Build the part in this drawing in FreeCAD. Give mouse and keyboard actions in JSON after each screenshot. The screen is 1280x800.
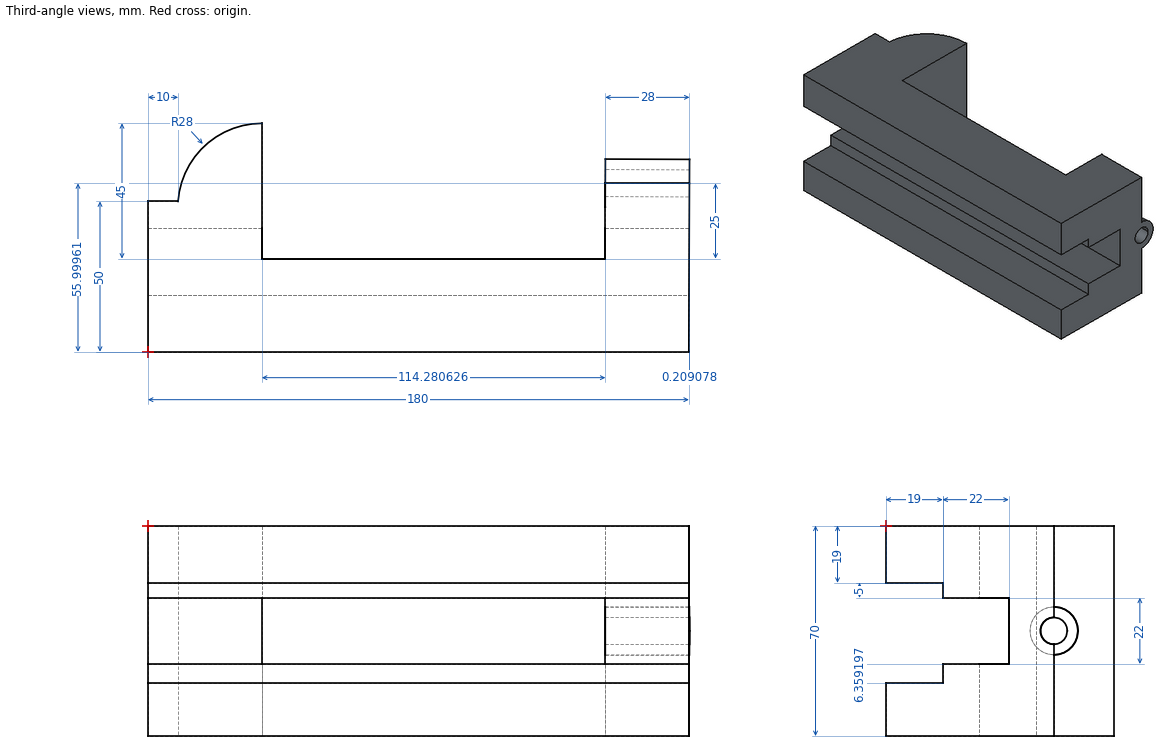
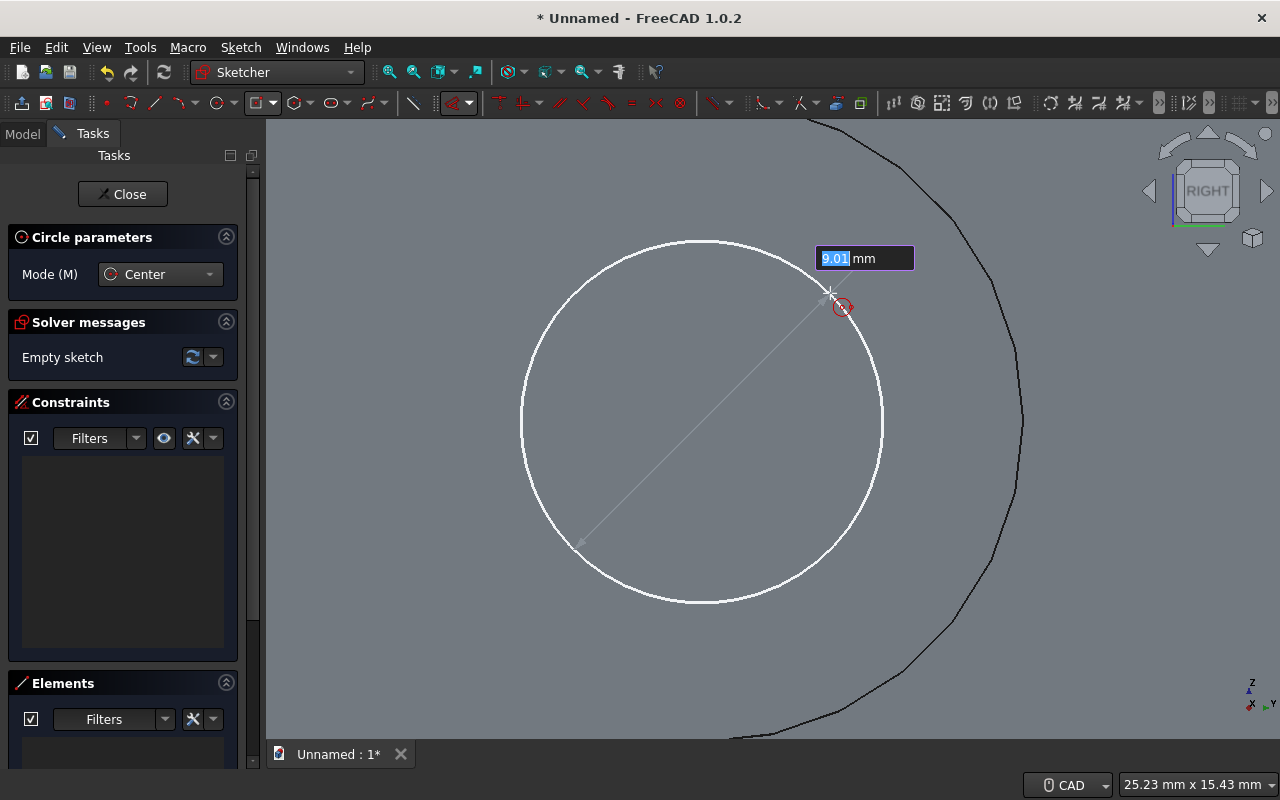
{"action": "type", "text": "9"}
{"action": "key", "text": "Return"}
{"action": "key", "text": "Escape"}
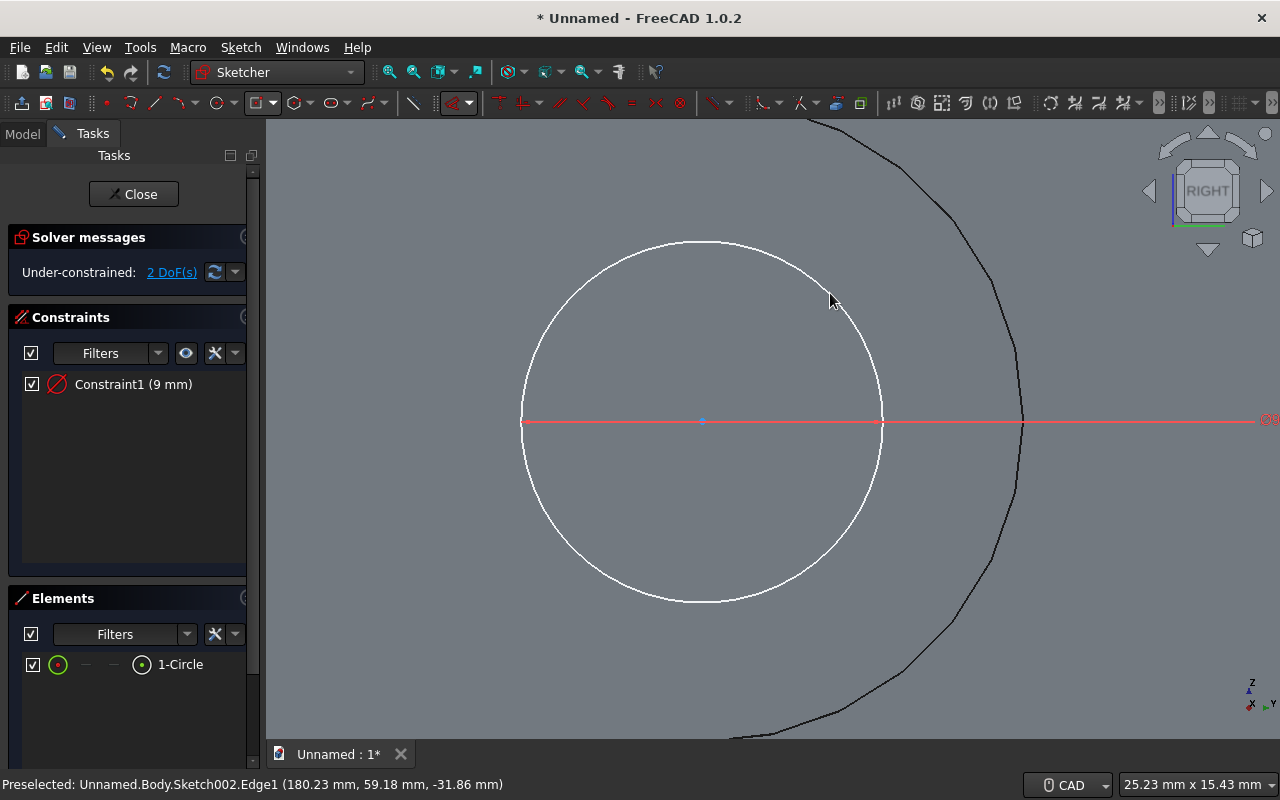
{"action": "left_click", "coordinate": [702, 422]}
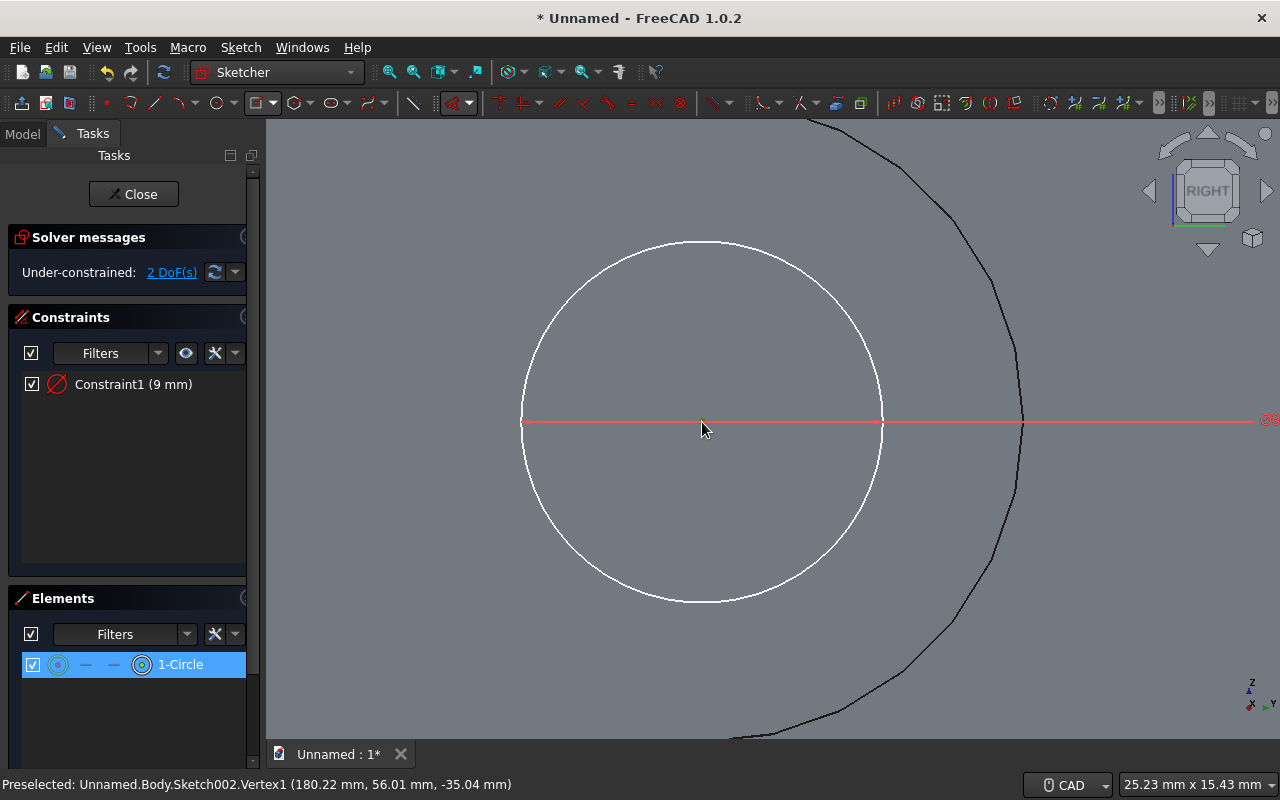
{"action": "key", "text": "i"}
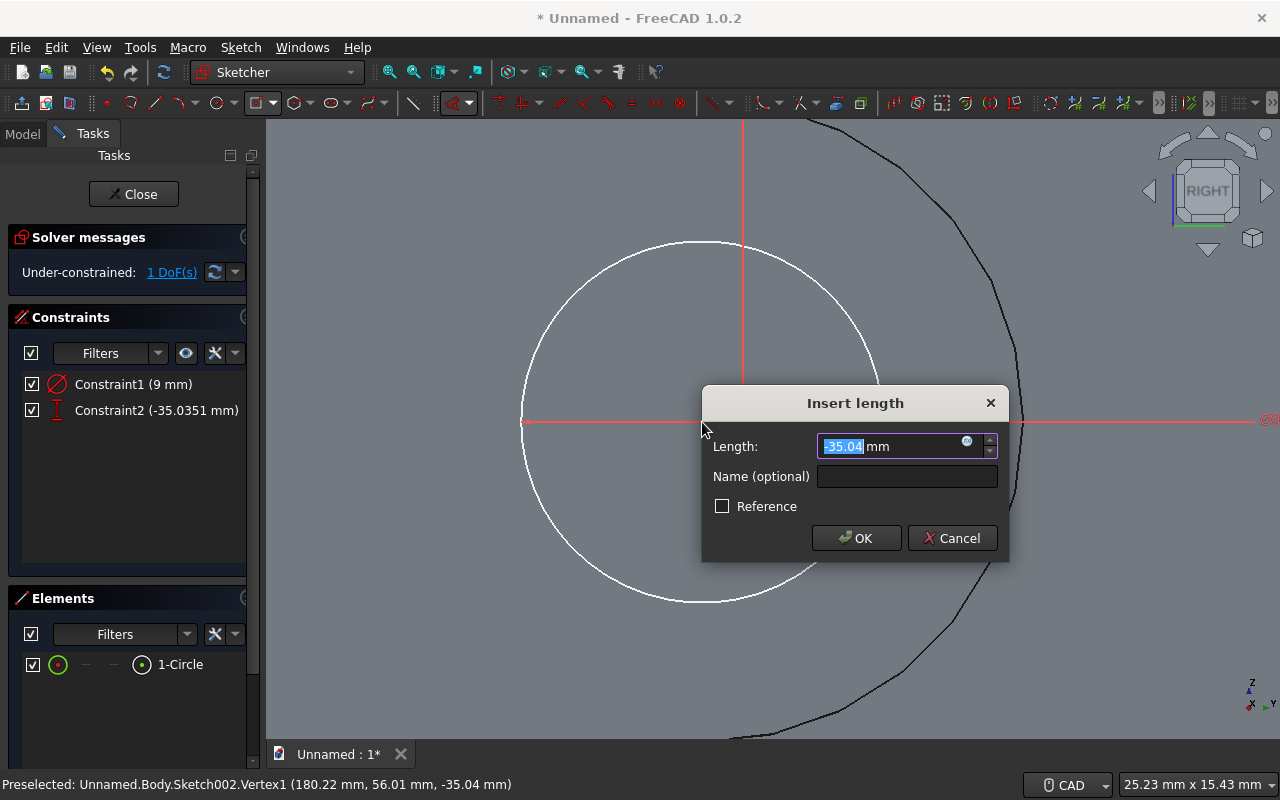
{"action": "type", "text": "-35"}
{"action": "key", "text": "Return"}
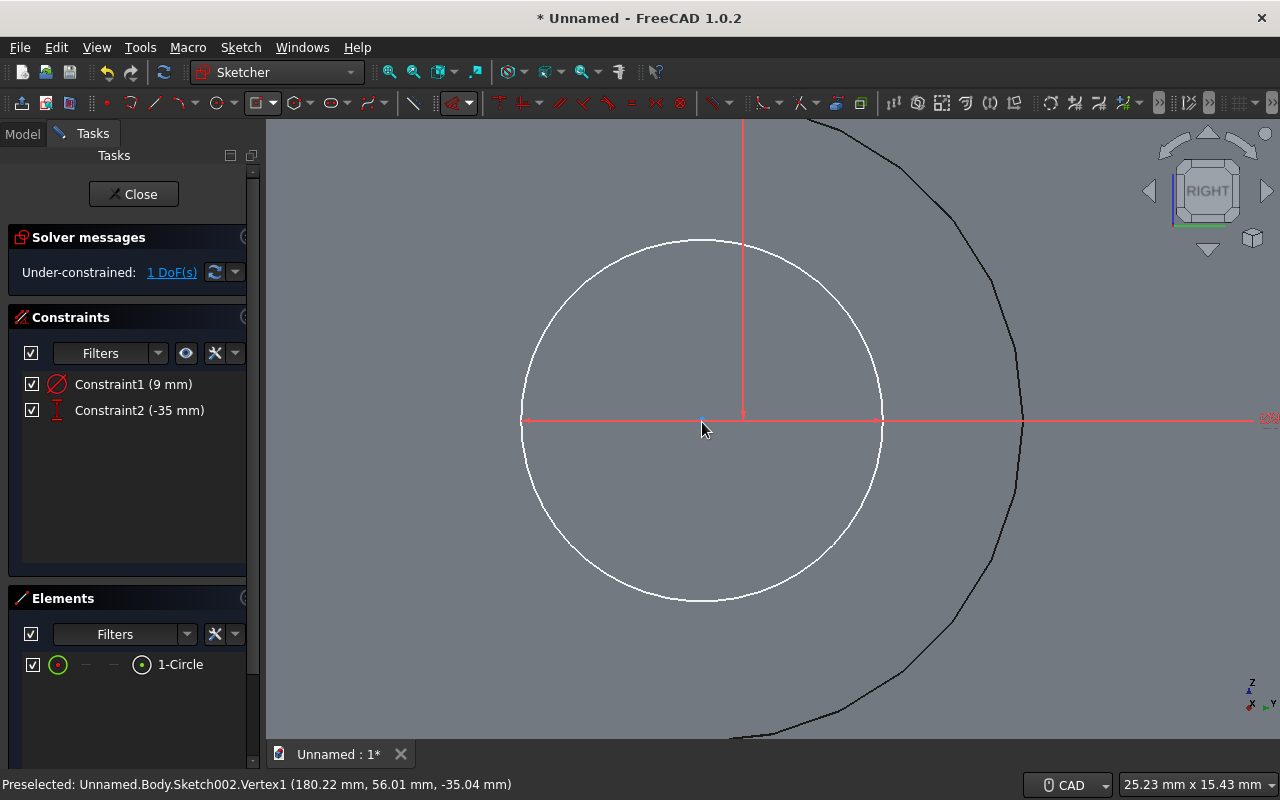
{"action": "left_click", "coordinate": [702, 421]}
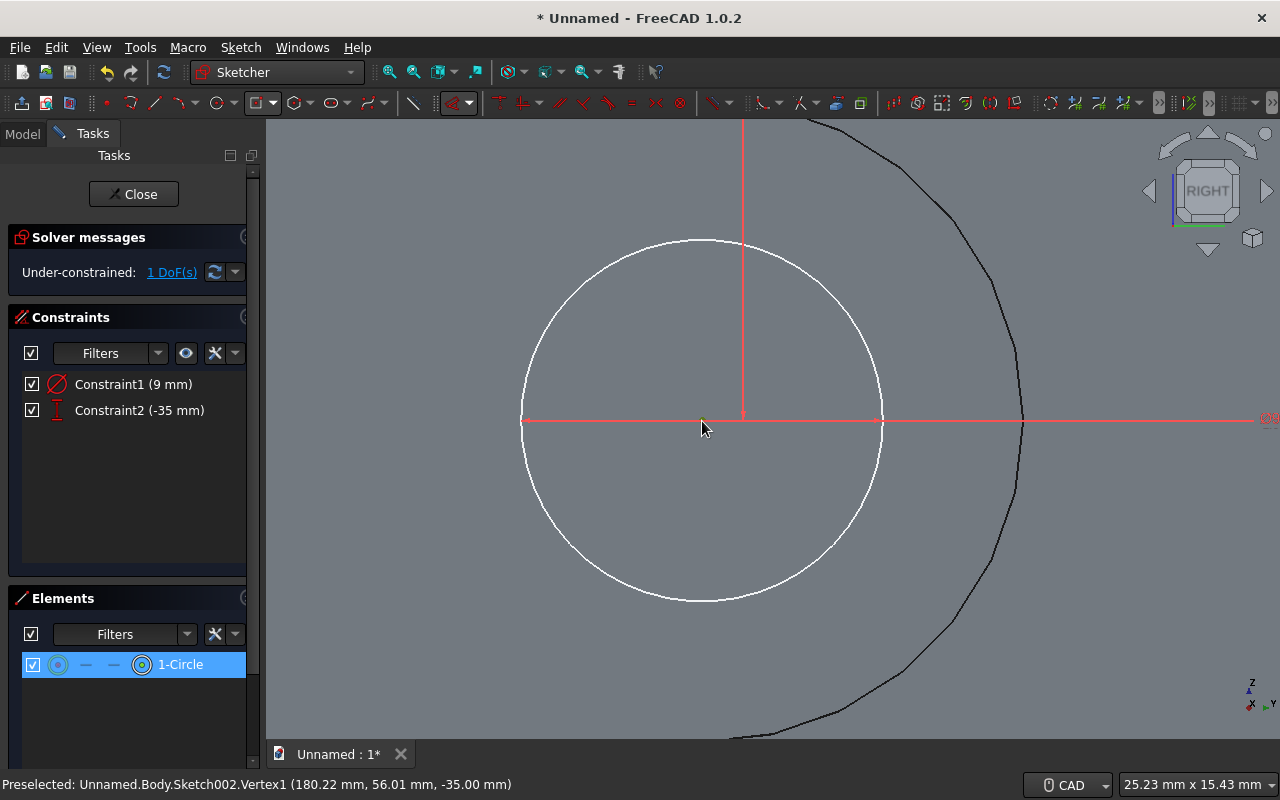
{"action": "left_click", "coordinate": [472, 104]}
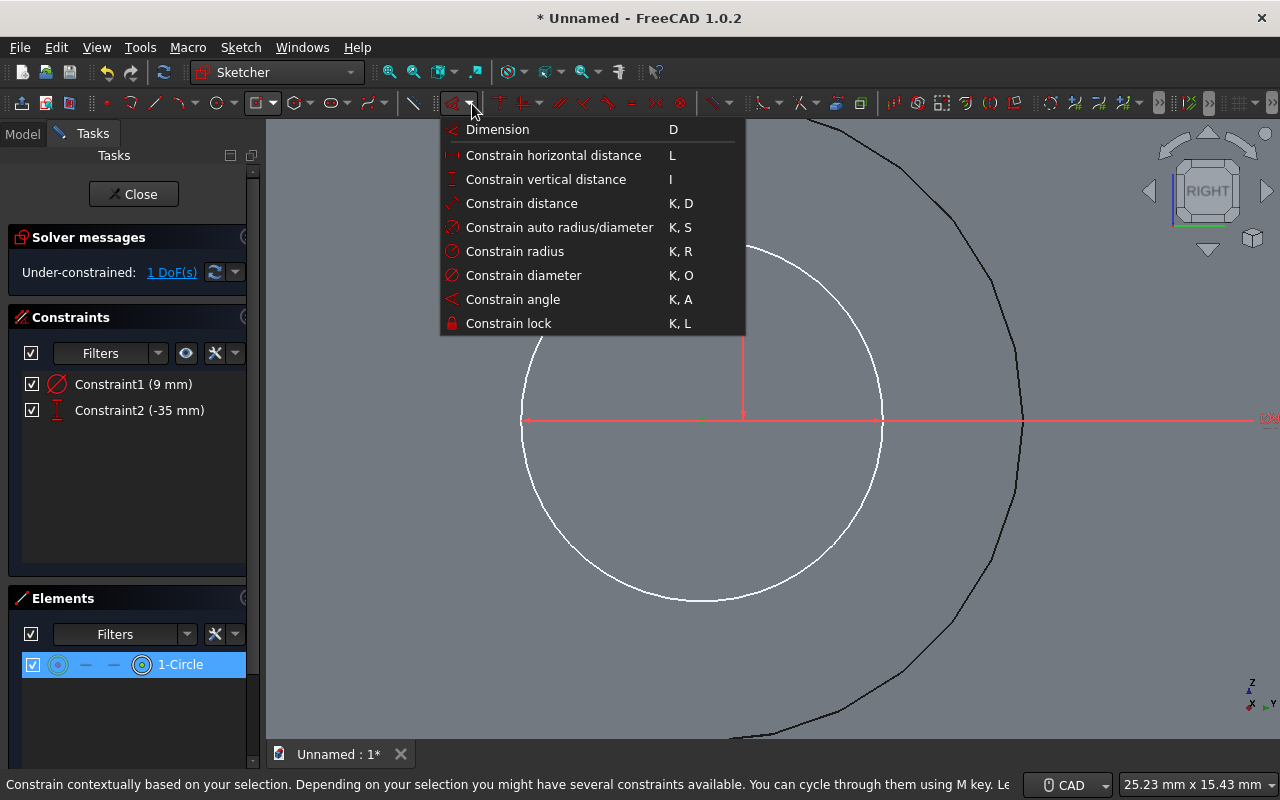
{"action": "left_click", "coordinate": [593, 155]}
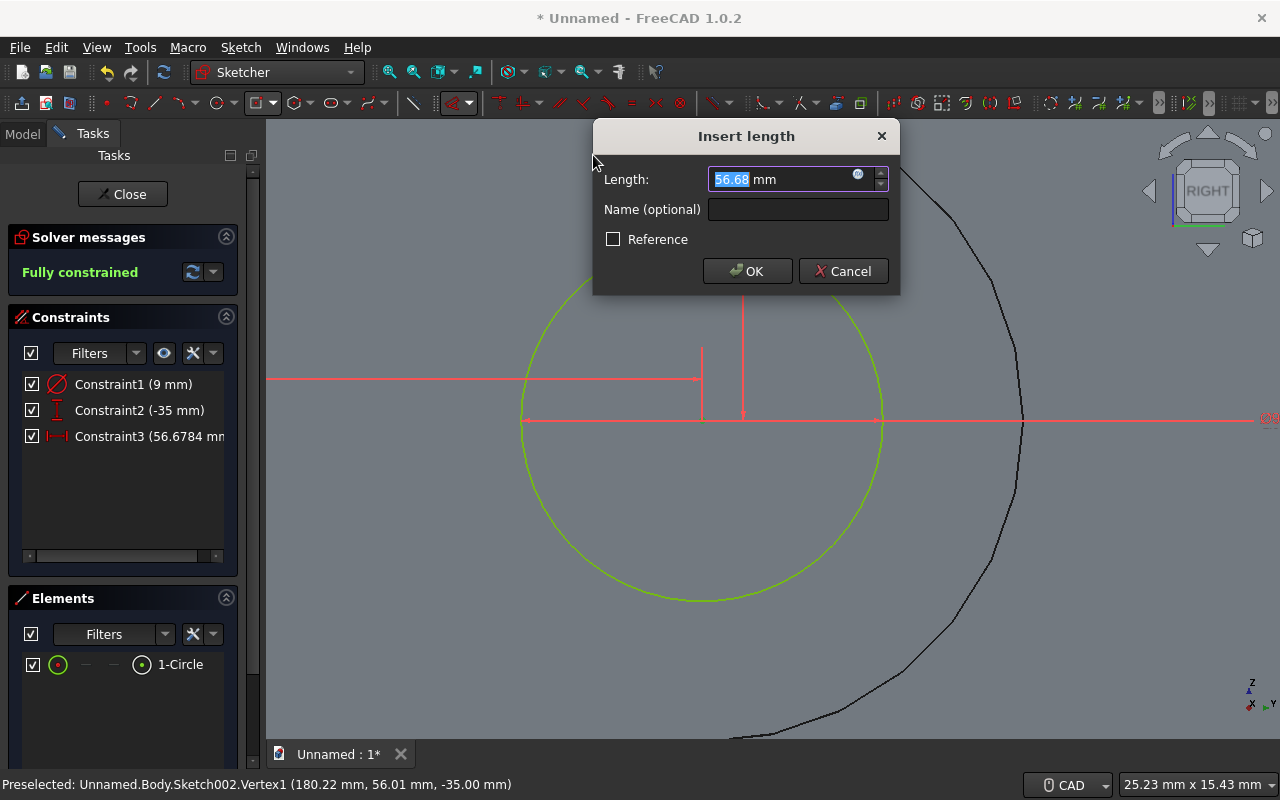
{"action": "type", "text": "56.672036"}
{"action": "key", "text": "Return"}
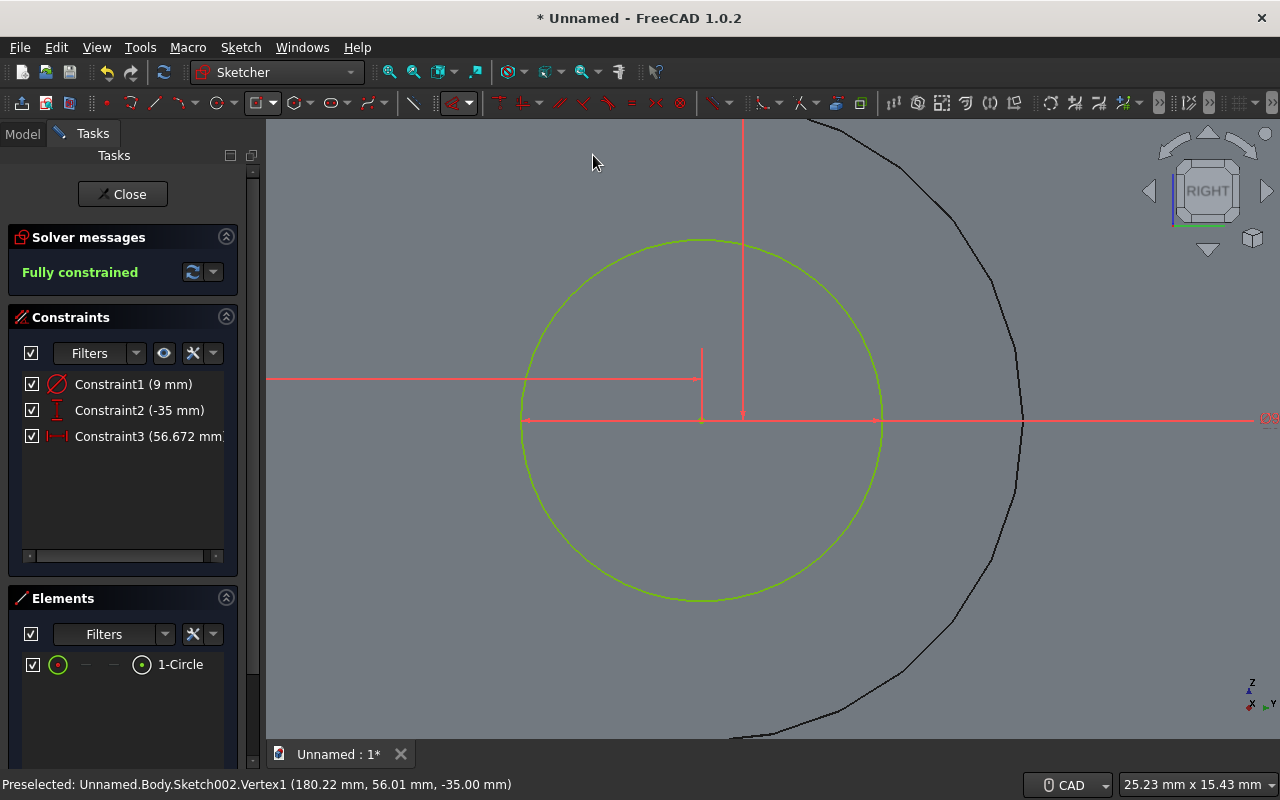
{"action": "left_click", "coordinate": [123, 194]}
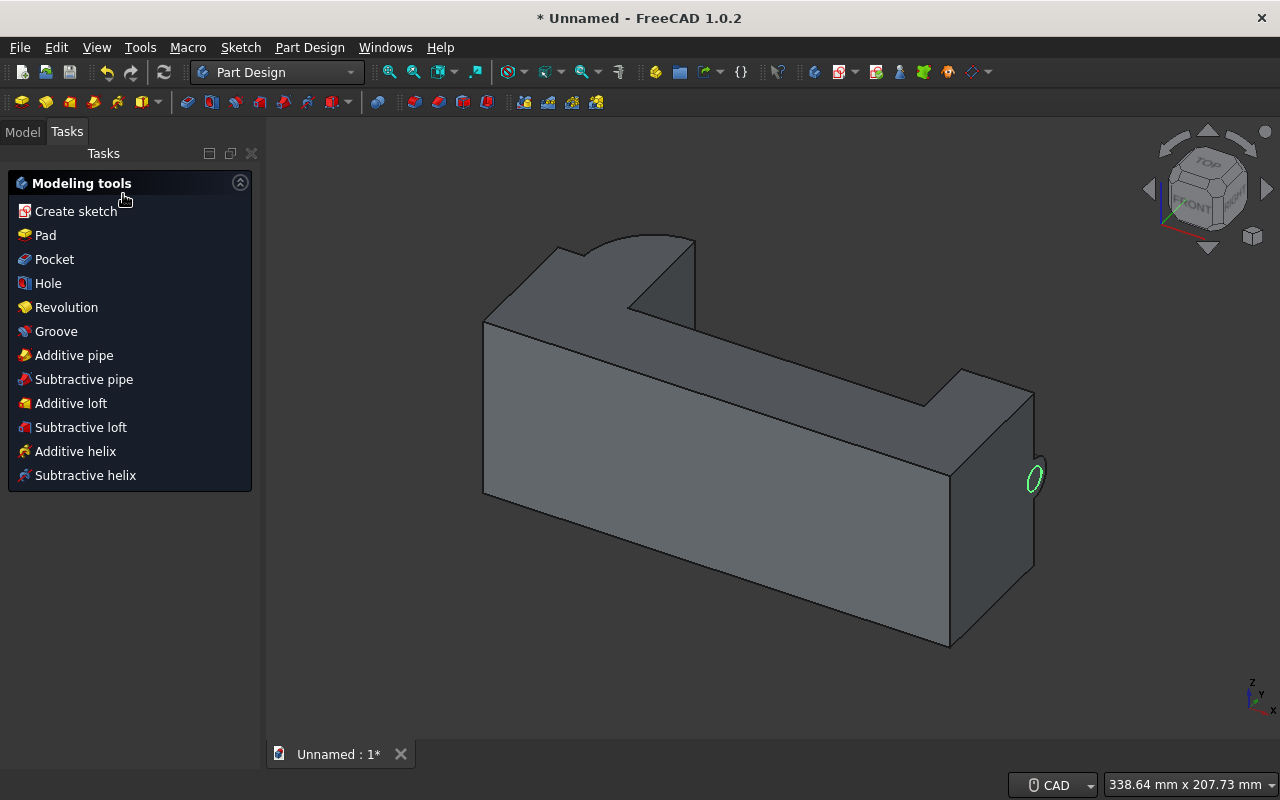
{"action": "left_click", "coordinate": [188, 102]}